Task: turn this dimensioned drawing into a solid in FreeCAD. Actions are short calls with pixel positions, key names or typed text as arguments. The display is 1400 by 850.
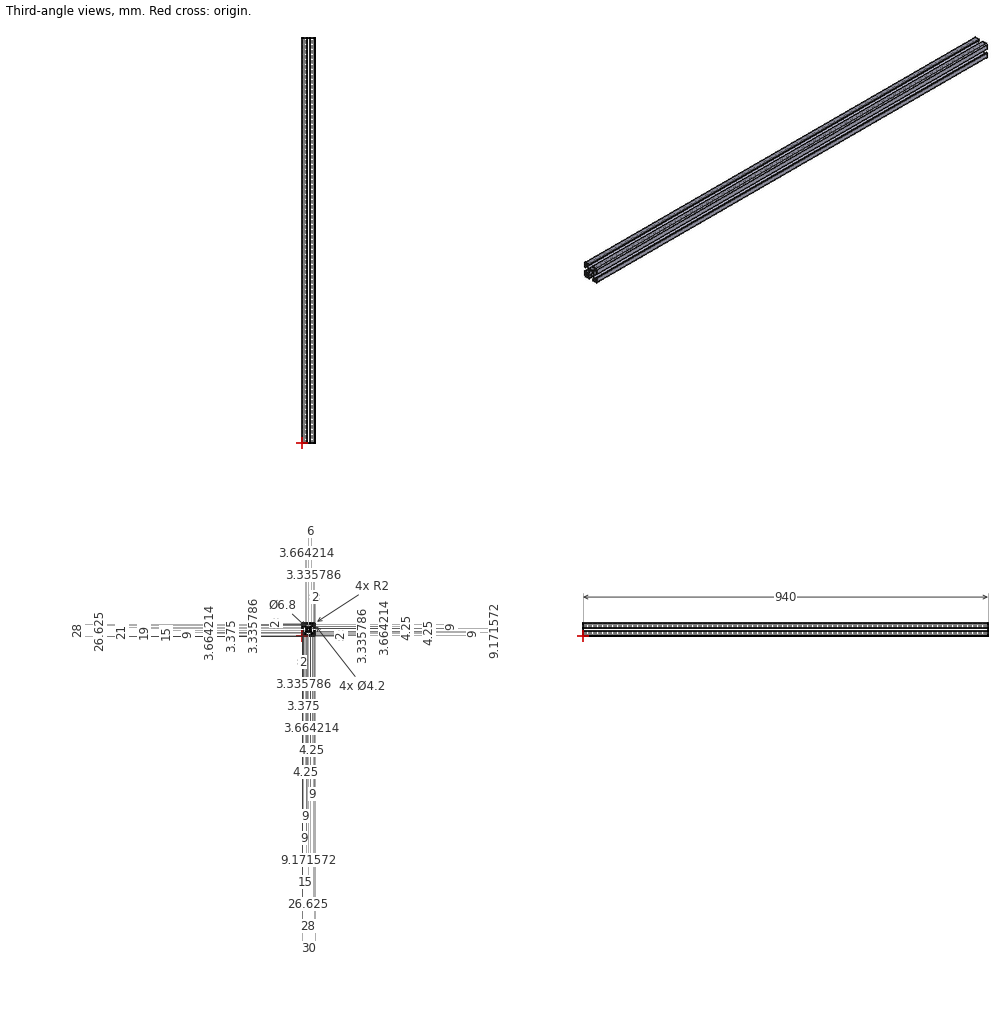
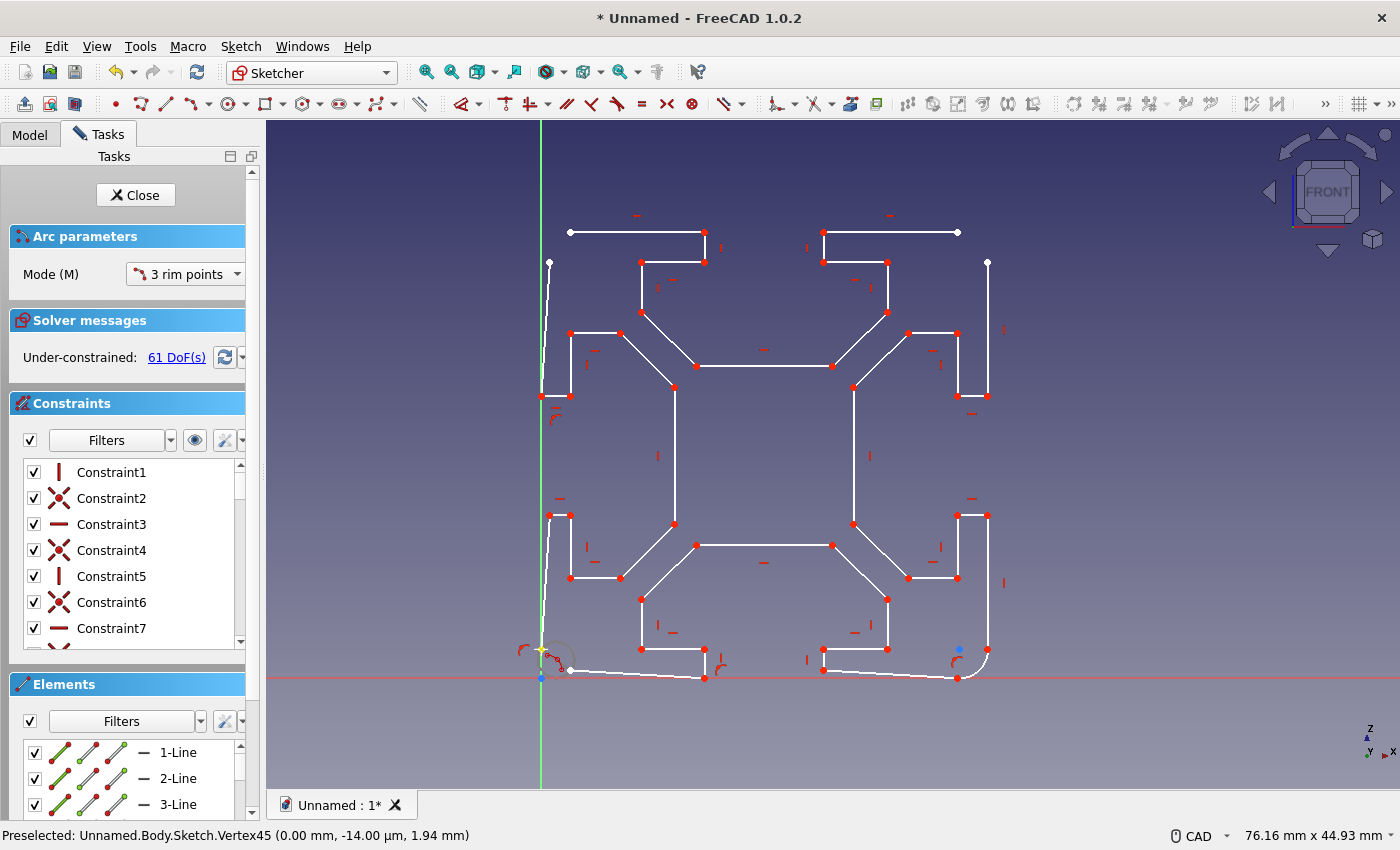
scroll(550, 670, up, 3)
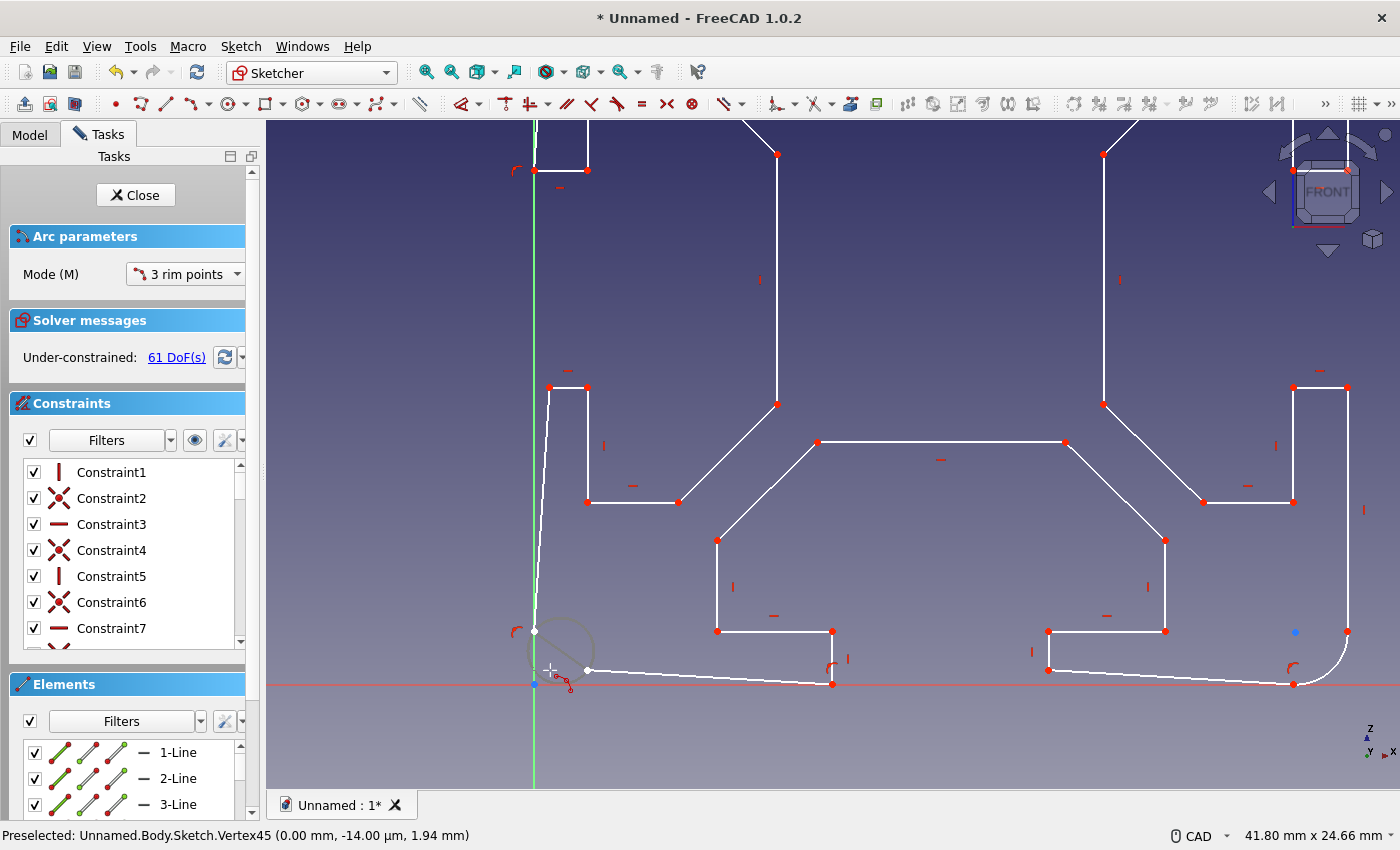
click(550, 669)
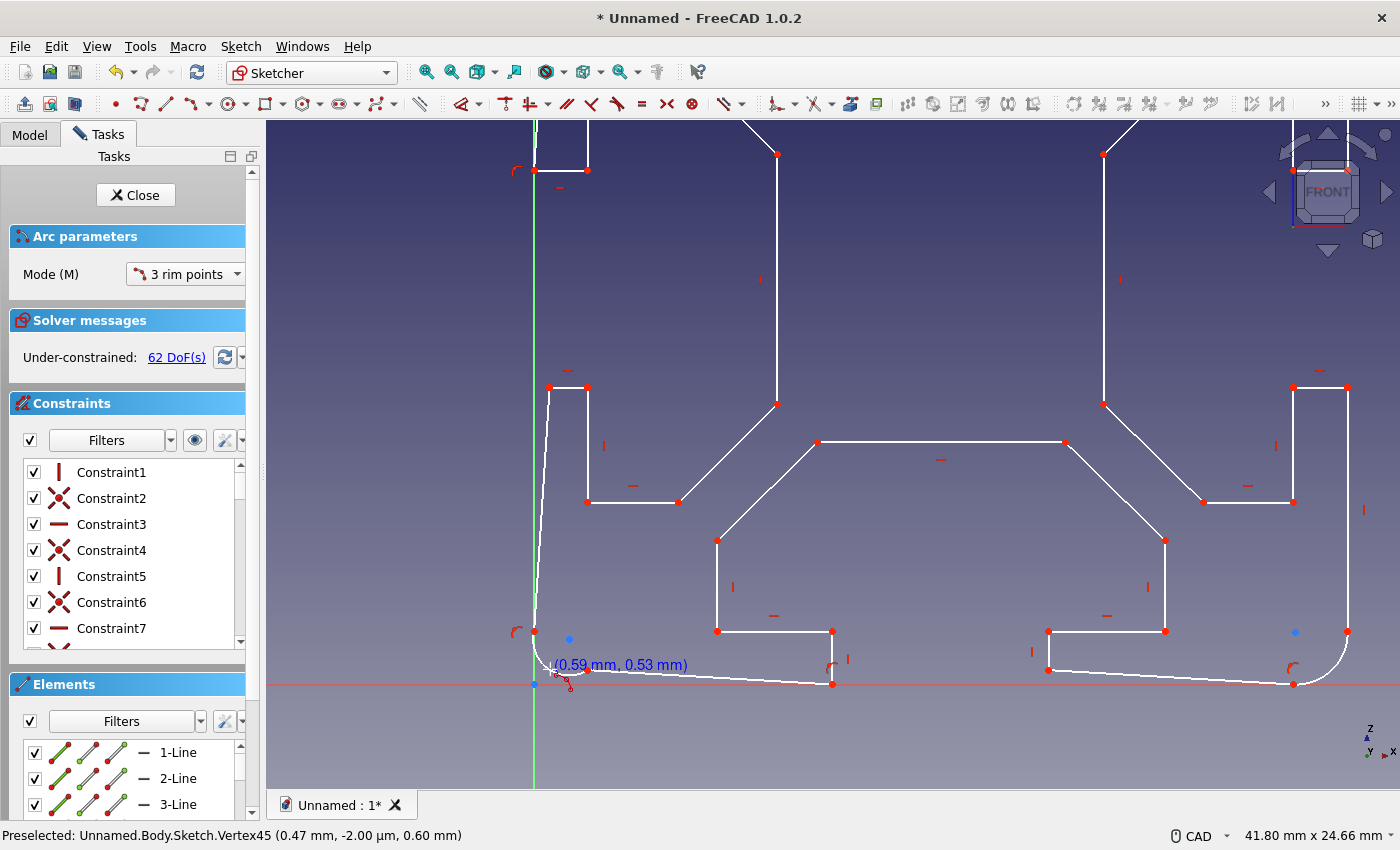
scroll(550, 670, down, 3)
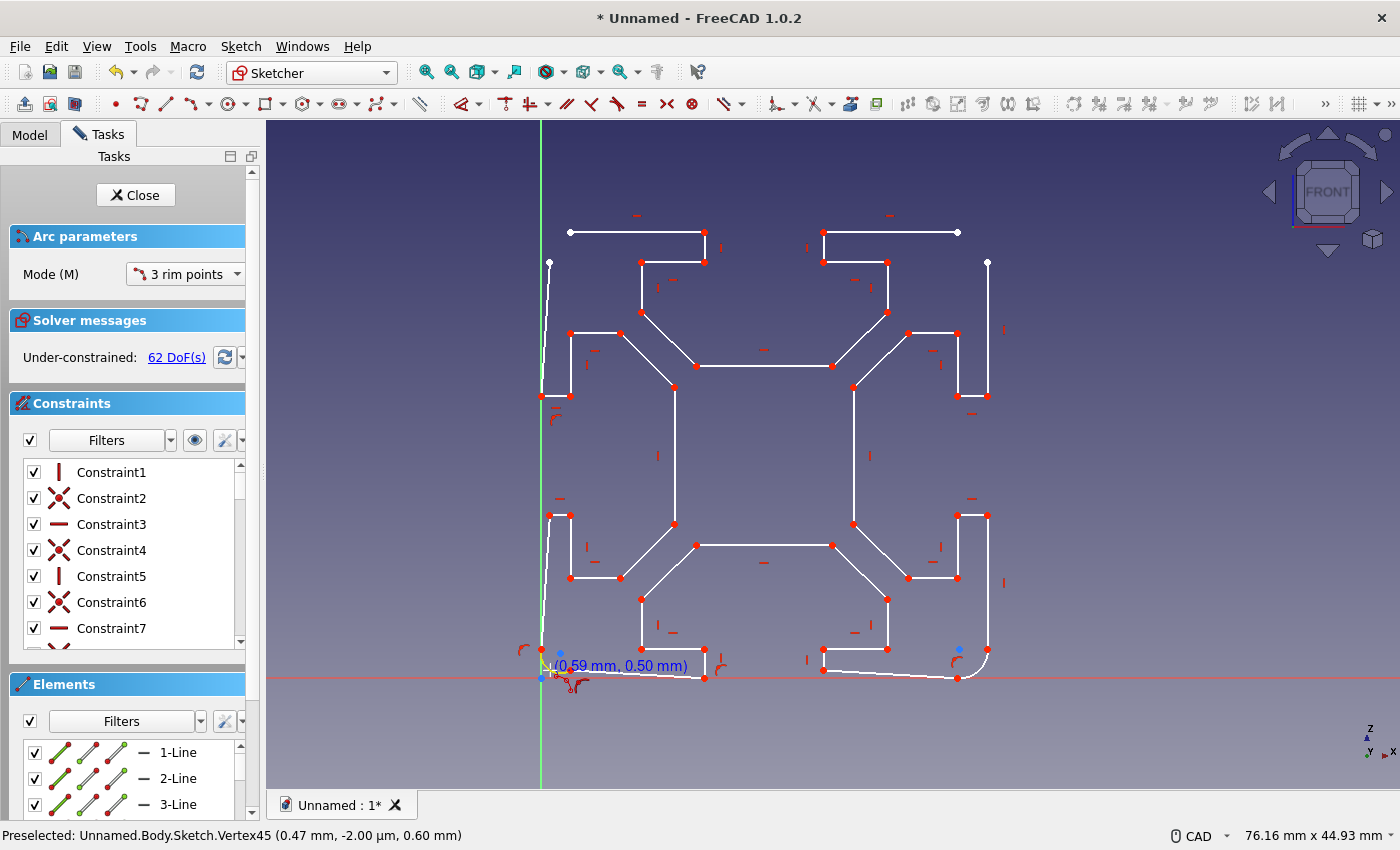
click(550, 262)
click(571, 232)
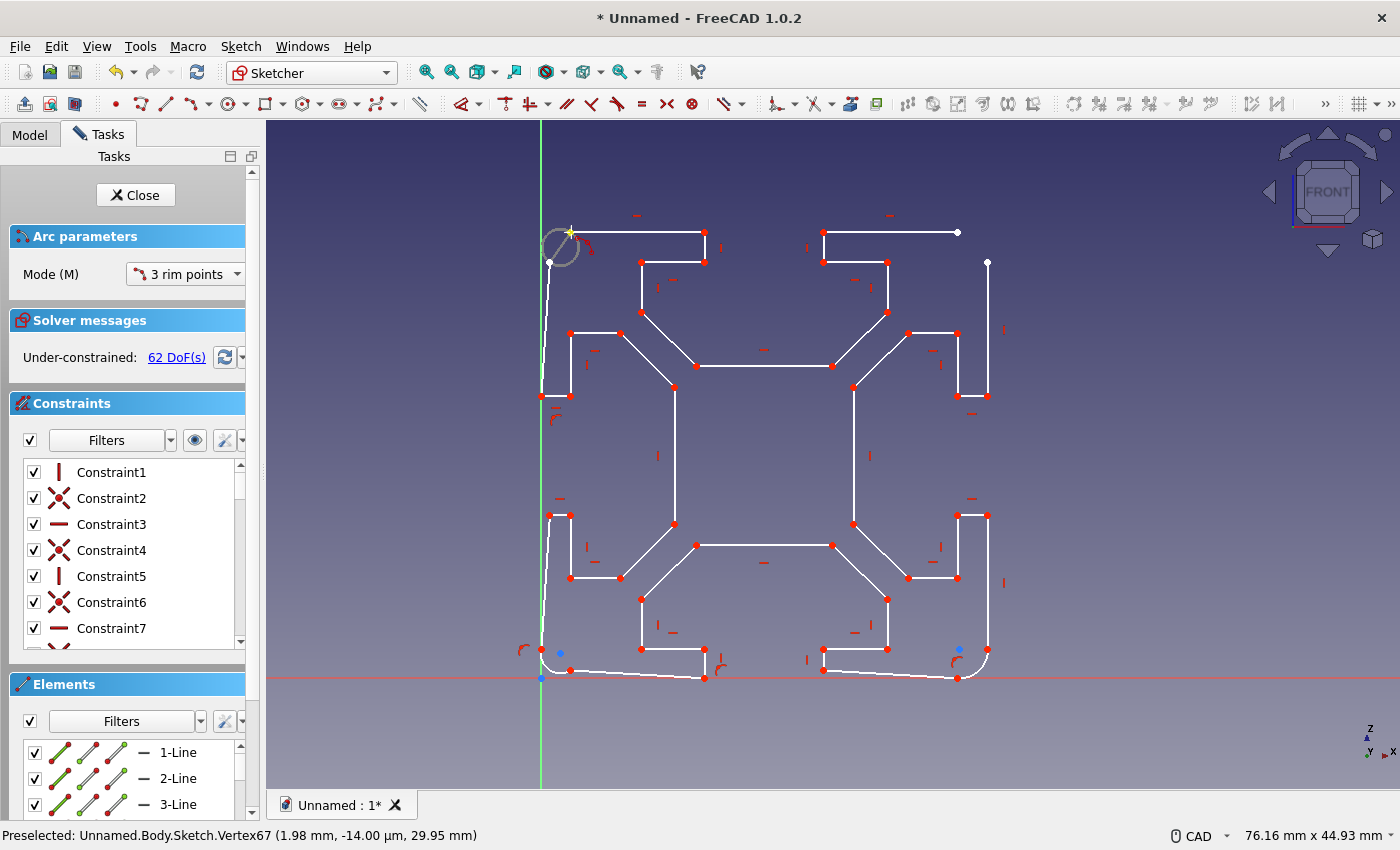
scroll(550, 240, up, 3)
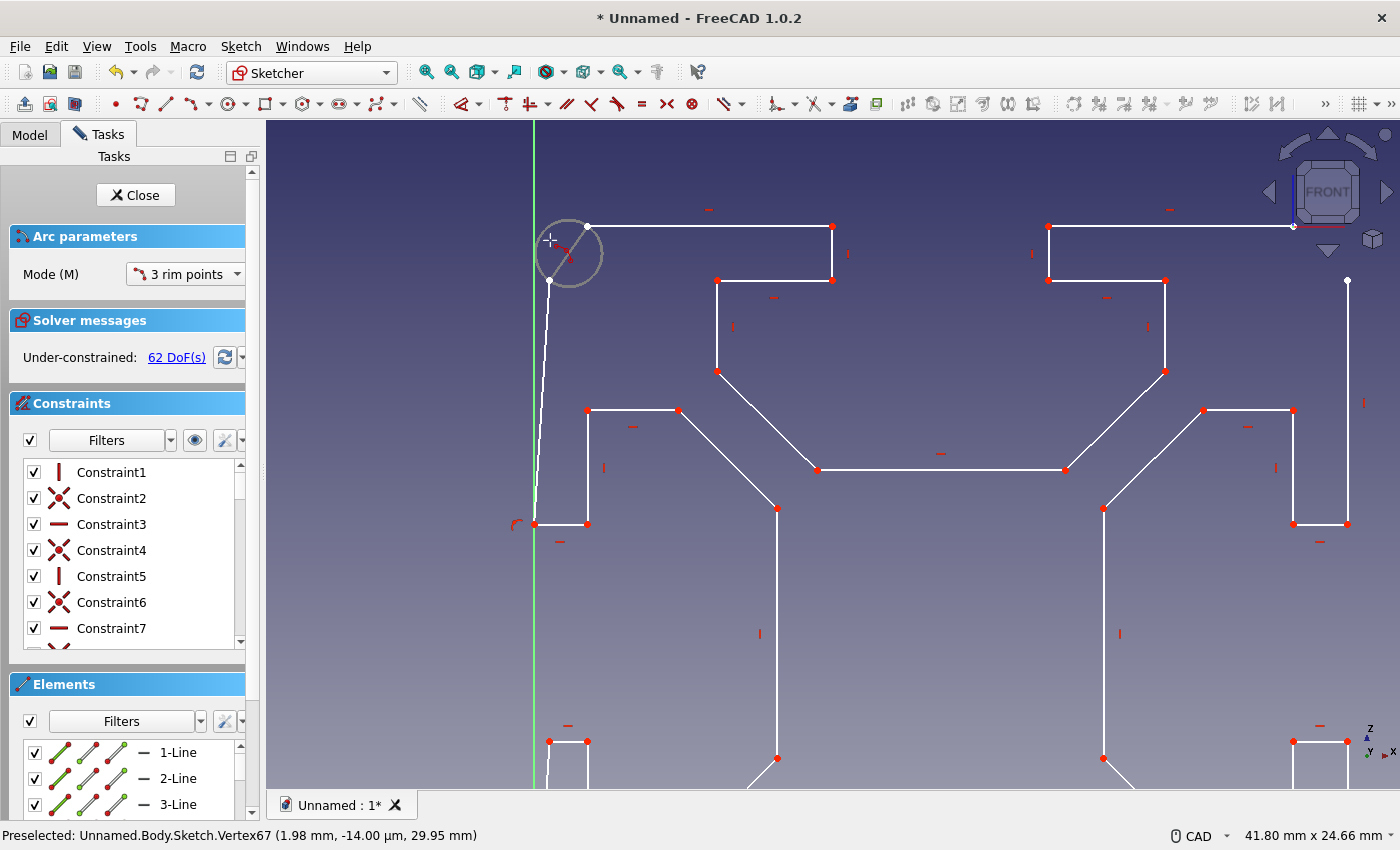
click(550, 241)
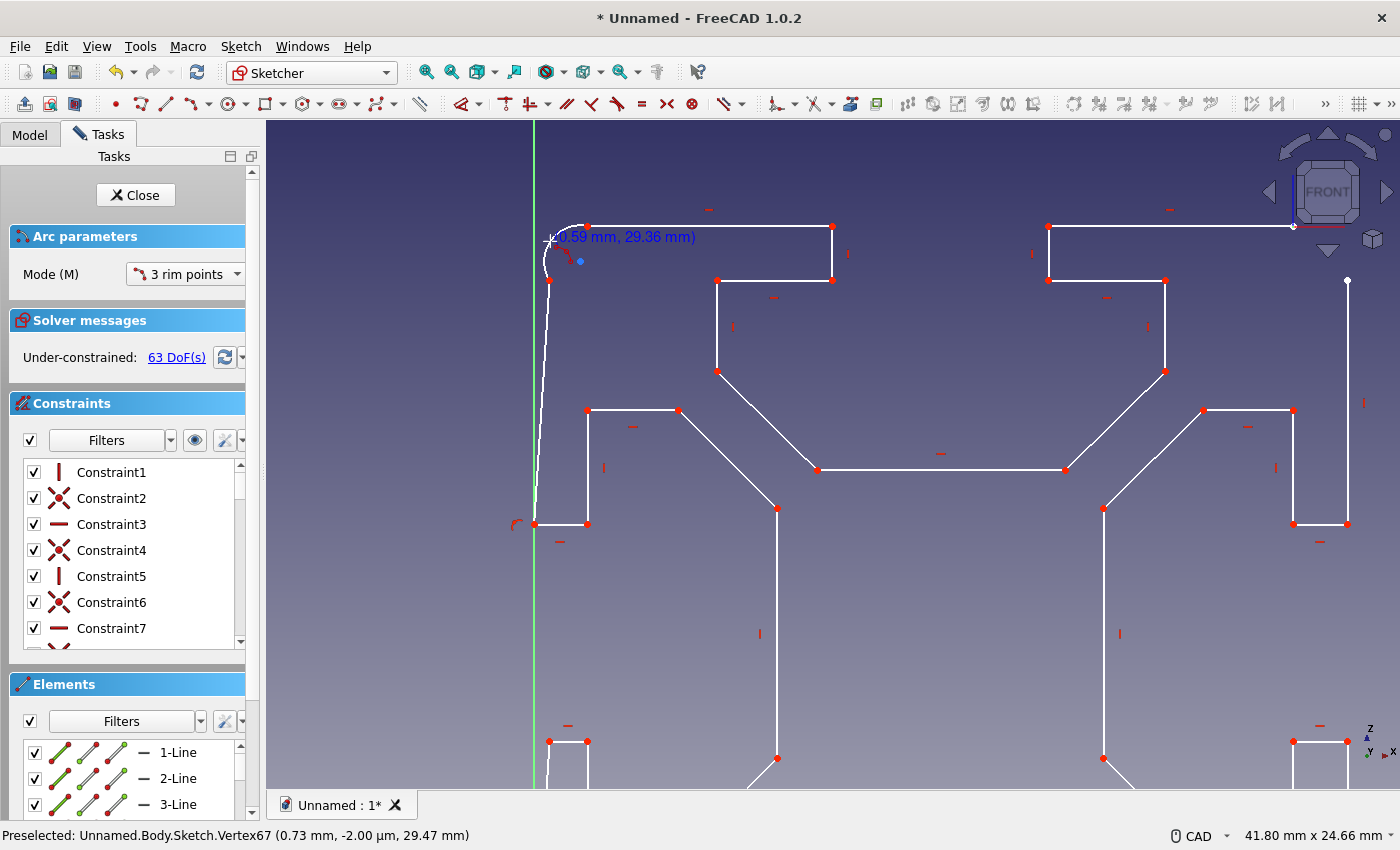
scroll(550, 239, down, 3)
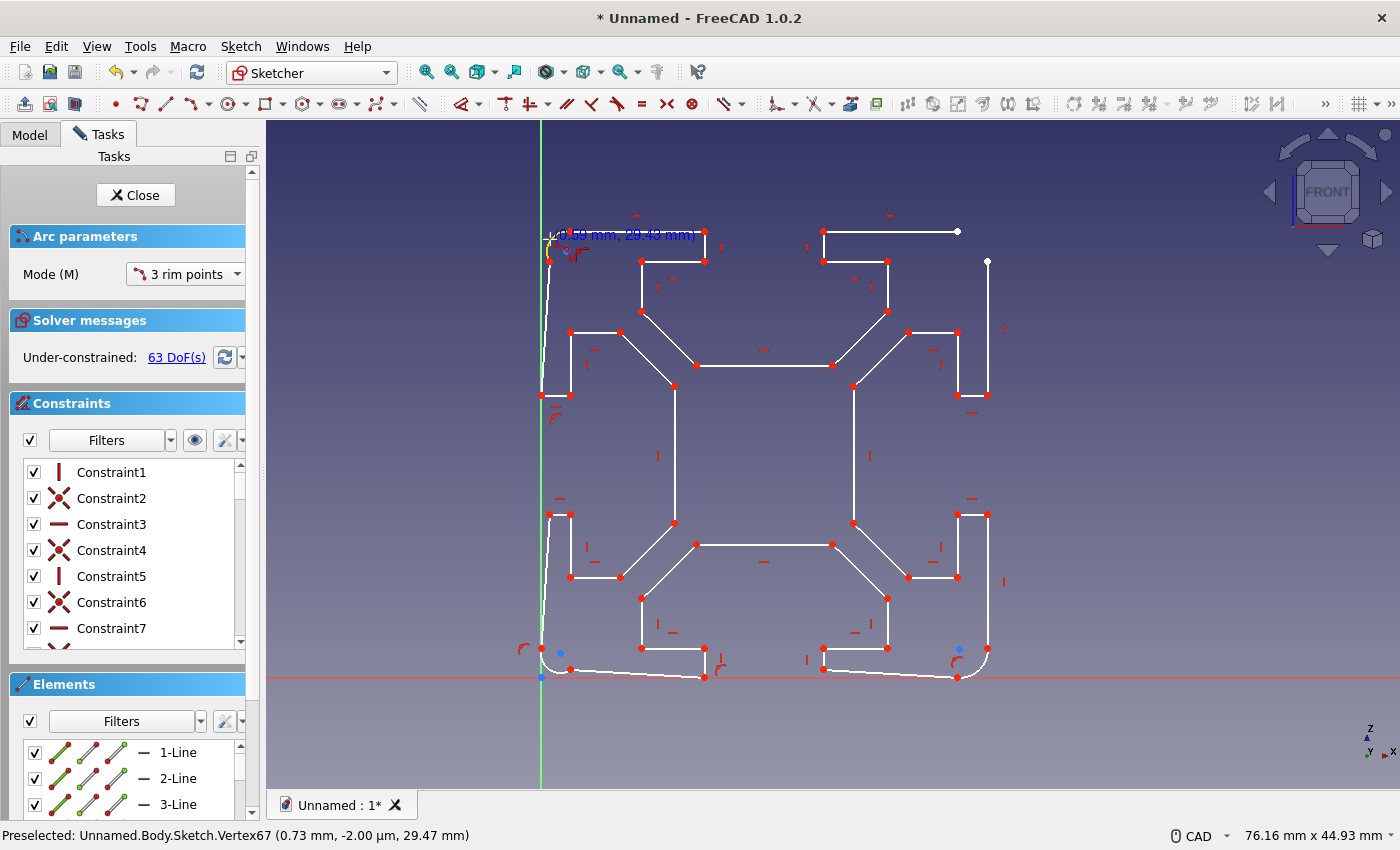
click(958, 232)
click(988, 262)